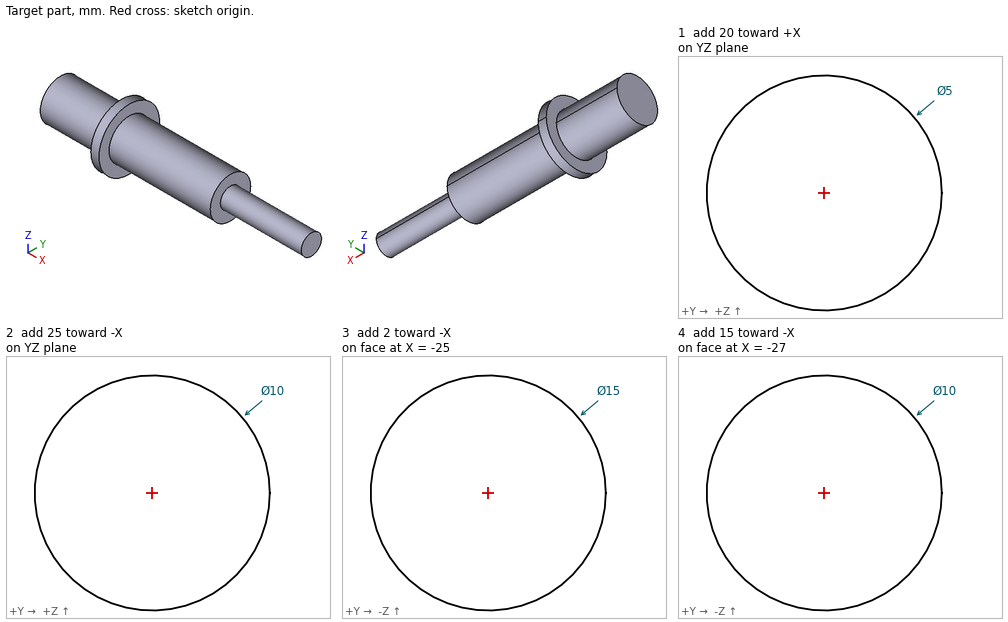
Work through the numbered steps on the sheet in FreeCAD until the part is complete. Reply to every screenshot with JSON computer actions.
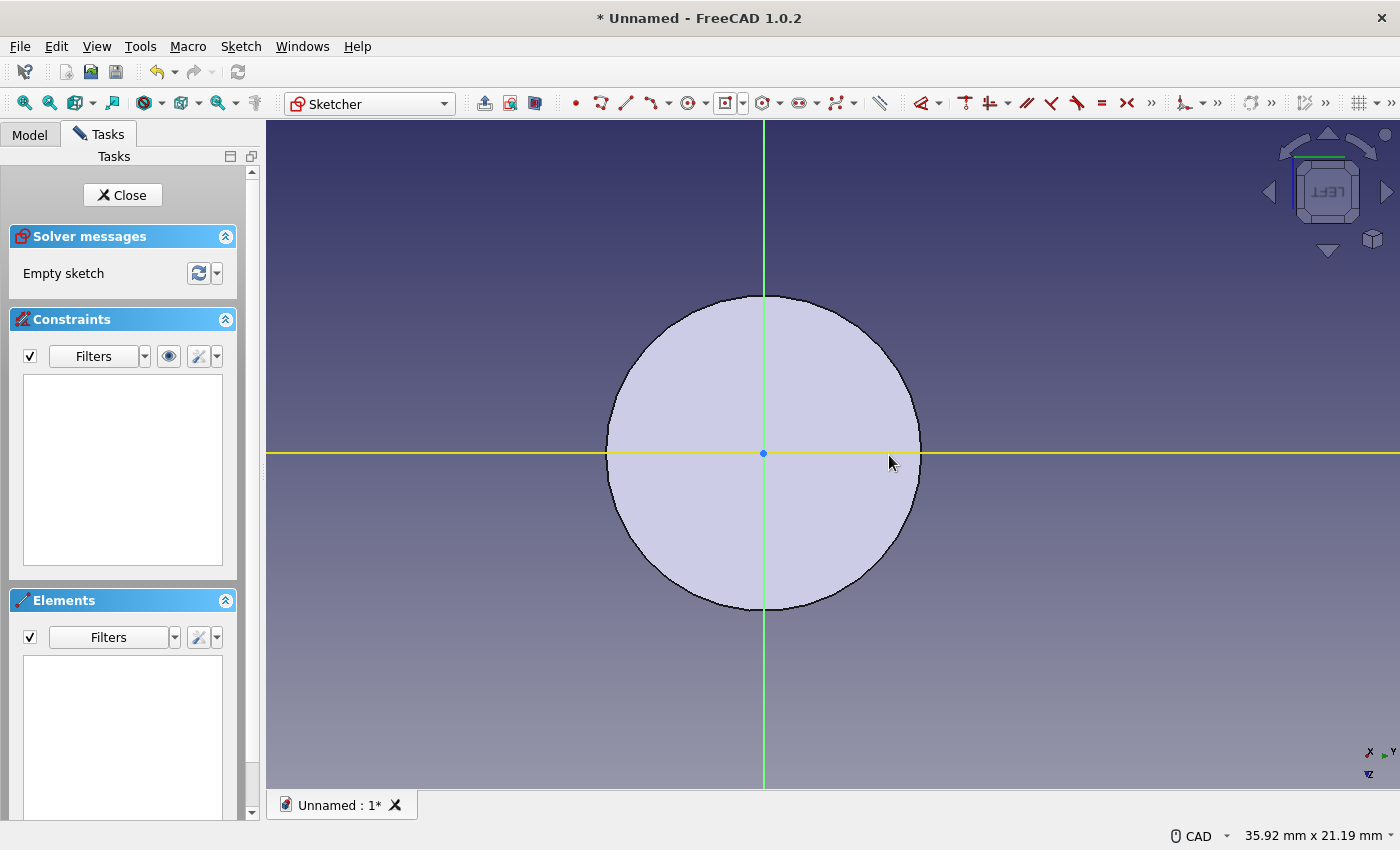
{"action": "key", "text": "g c"}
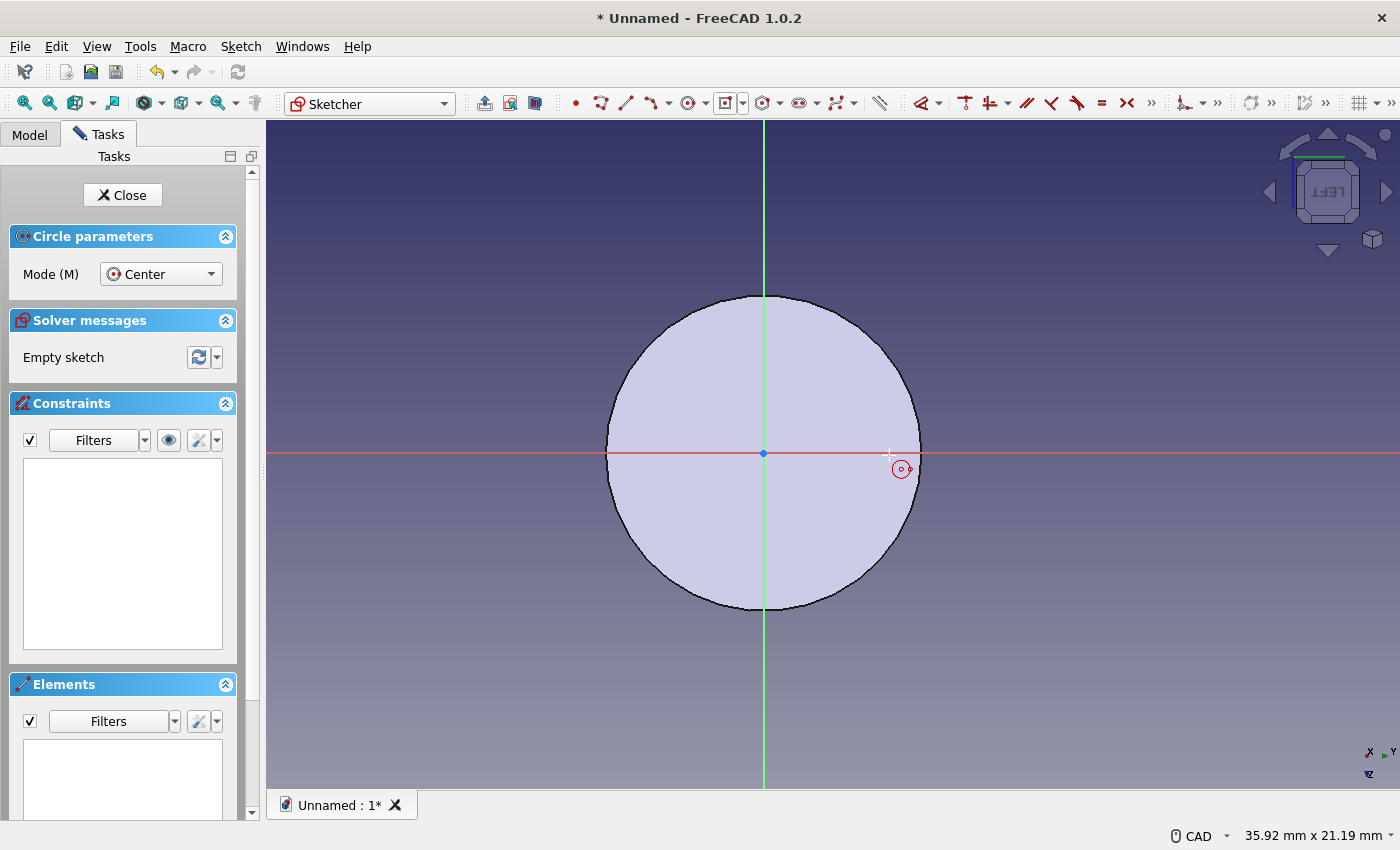
{"action": "left_click", "coordinate": [764, 453]}
{"action": "left_click", "coordinate": [931, 286]}
{"action": "key", "text": "Escape"}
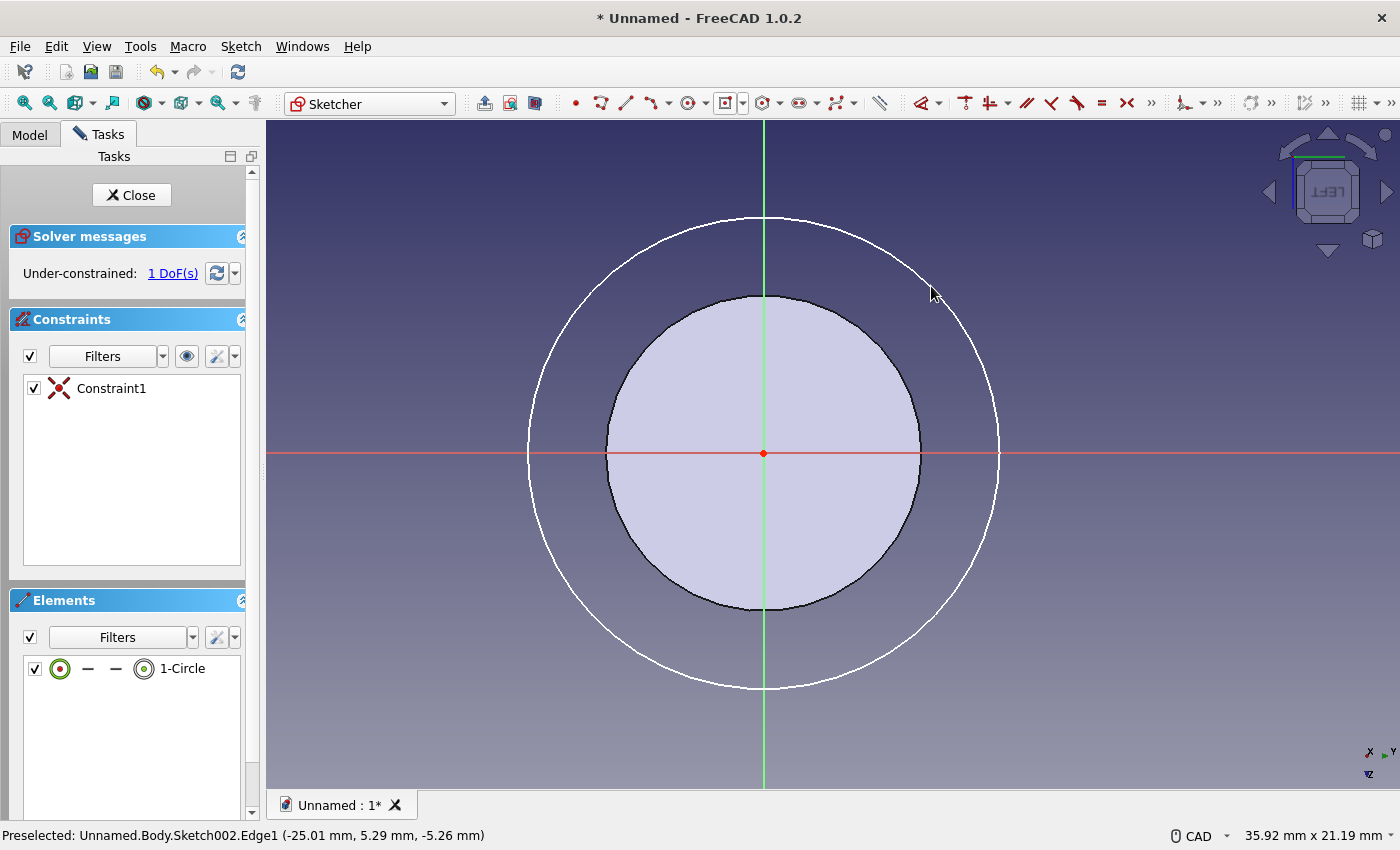
{"action": "key", "text": "d"}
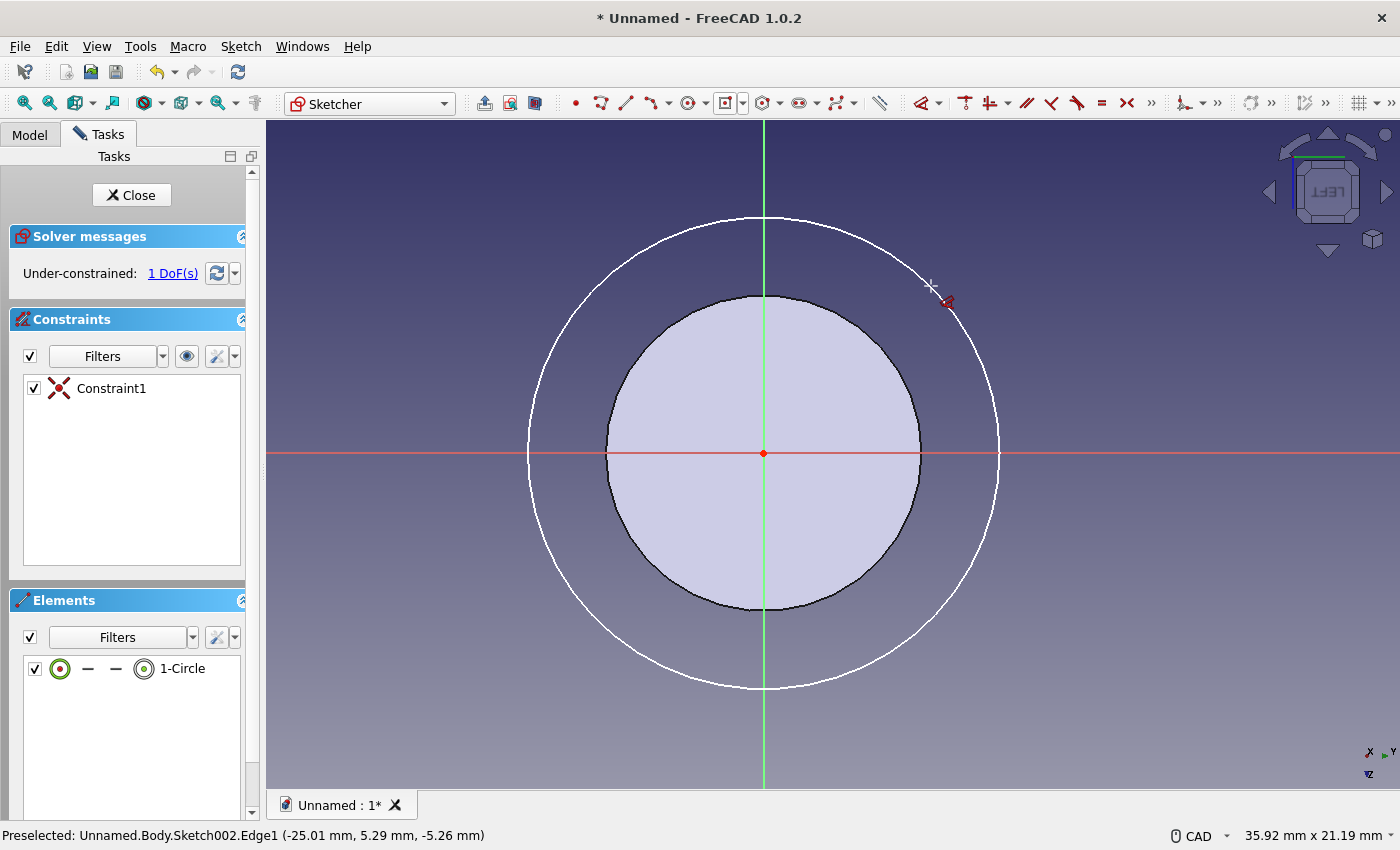
{"action": "left_click", "coordinate": [930, 286]}
{"action": "left_click", "coordinate": [953, 263]}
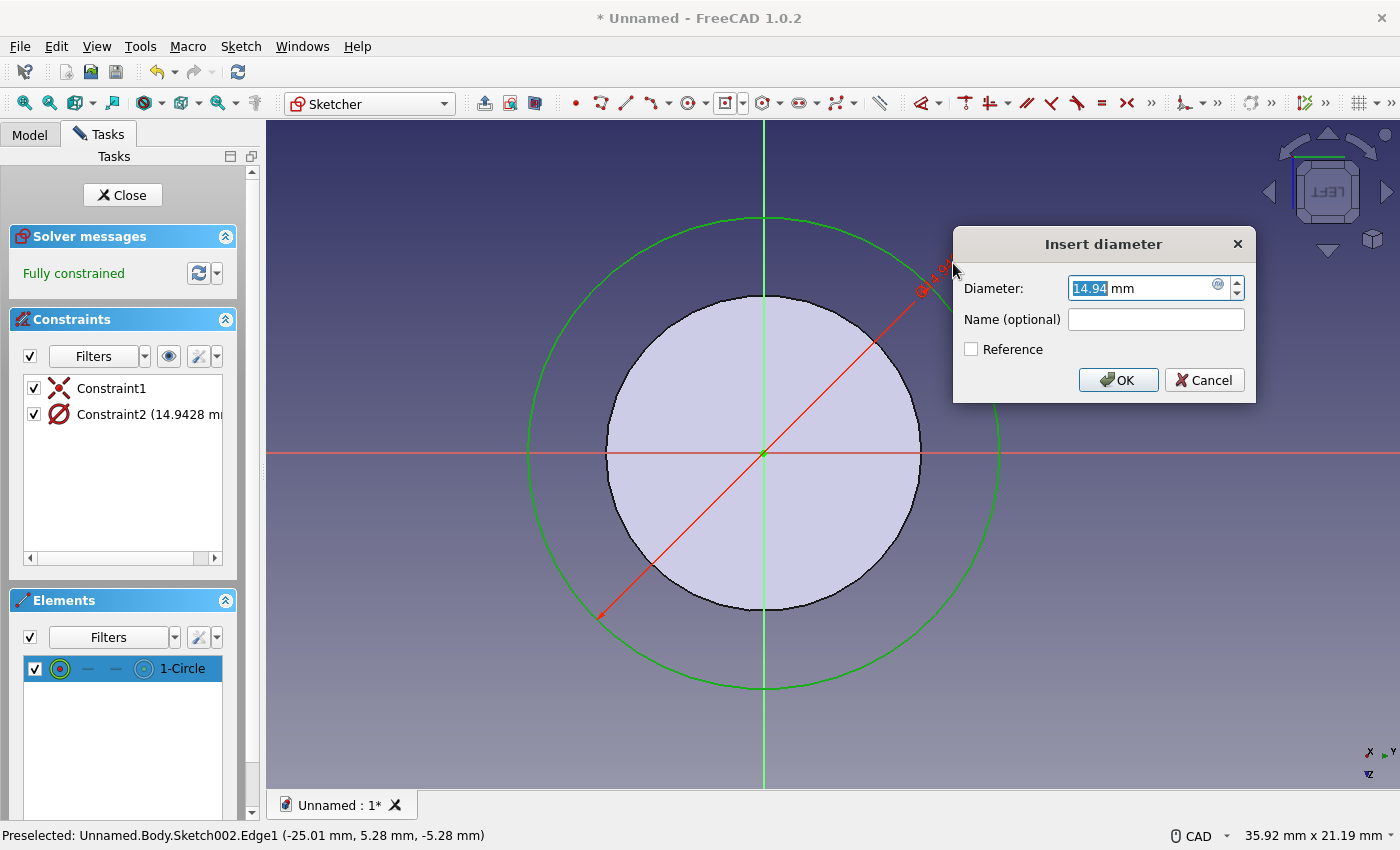
{"action": "type", "text": "15"}
{"action": "key", "text": "Return"}
{"action": "key", "text": "Escape"}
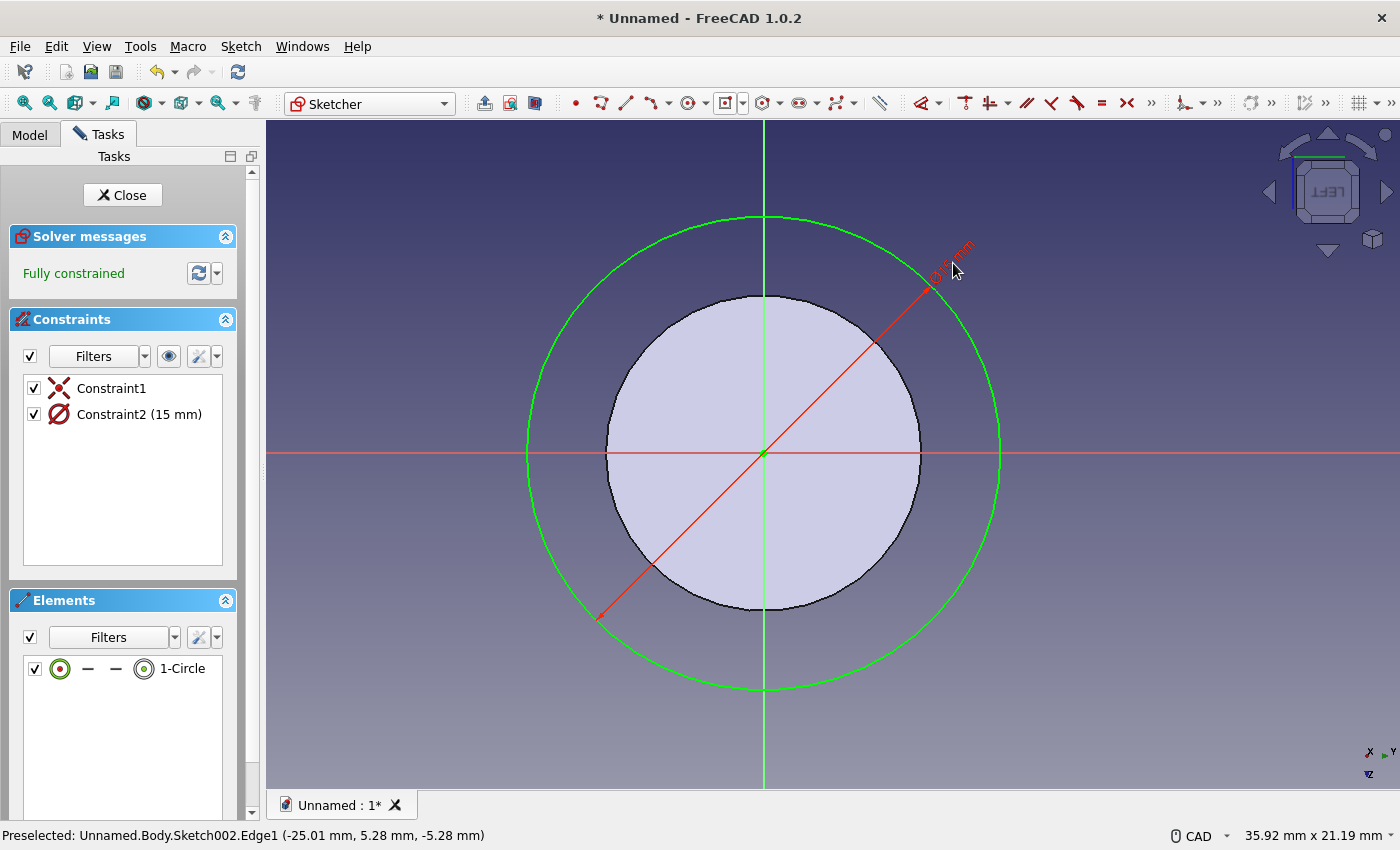
{"action": "left_click", "coordinate": [123, 195]}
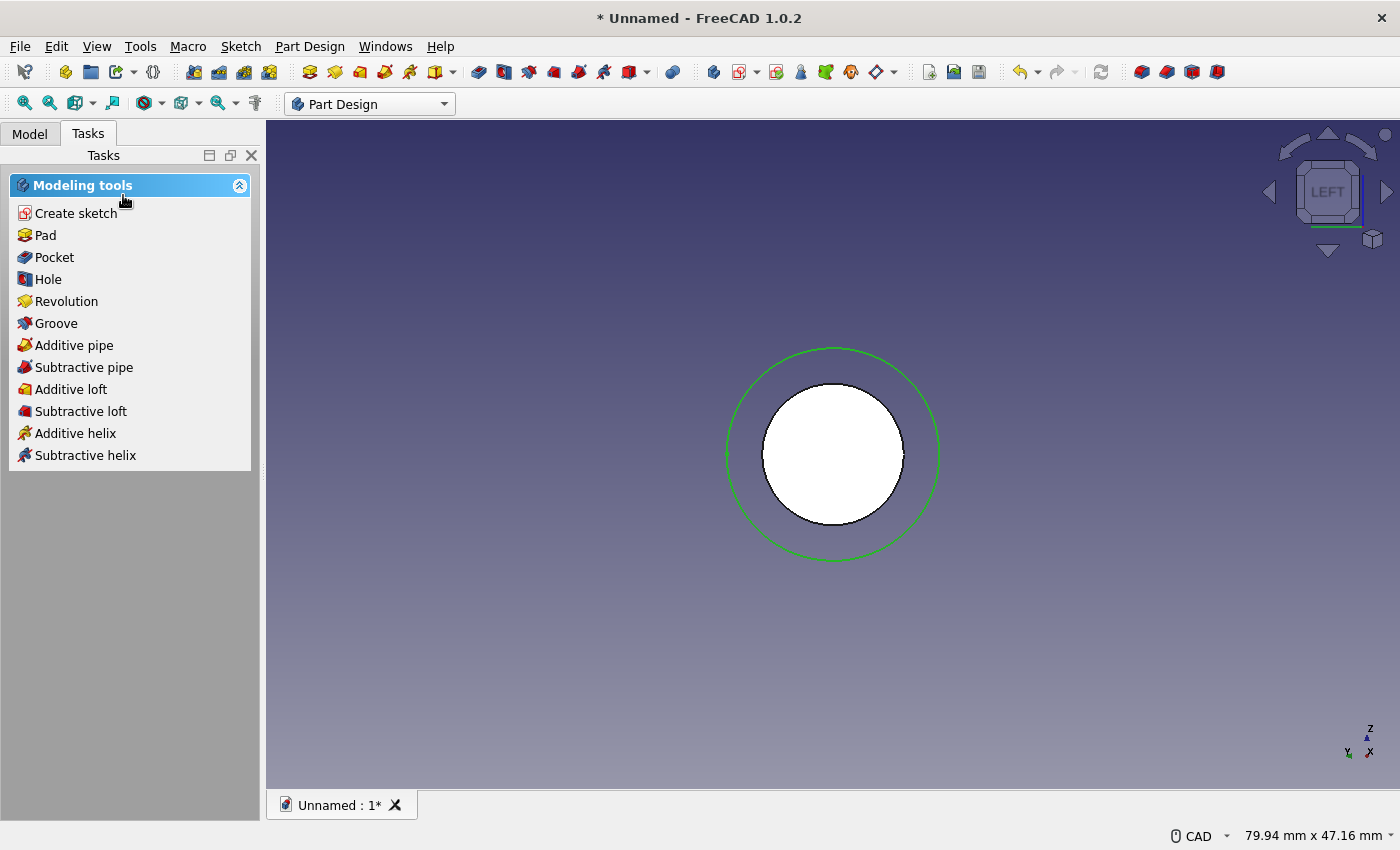
{"action": "left_click", "coordinate": [310, 72]}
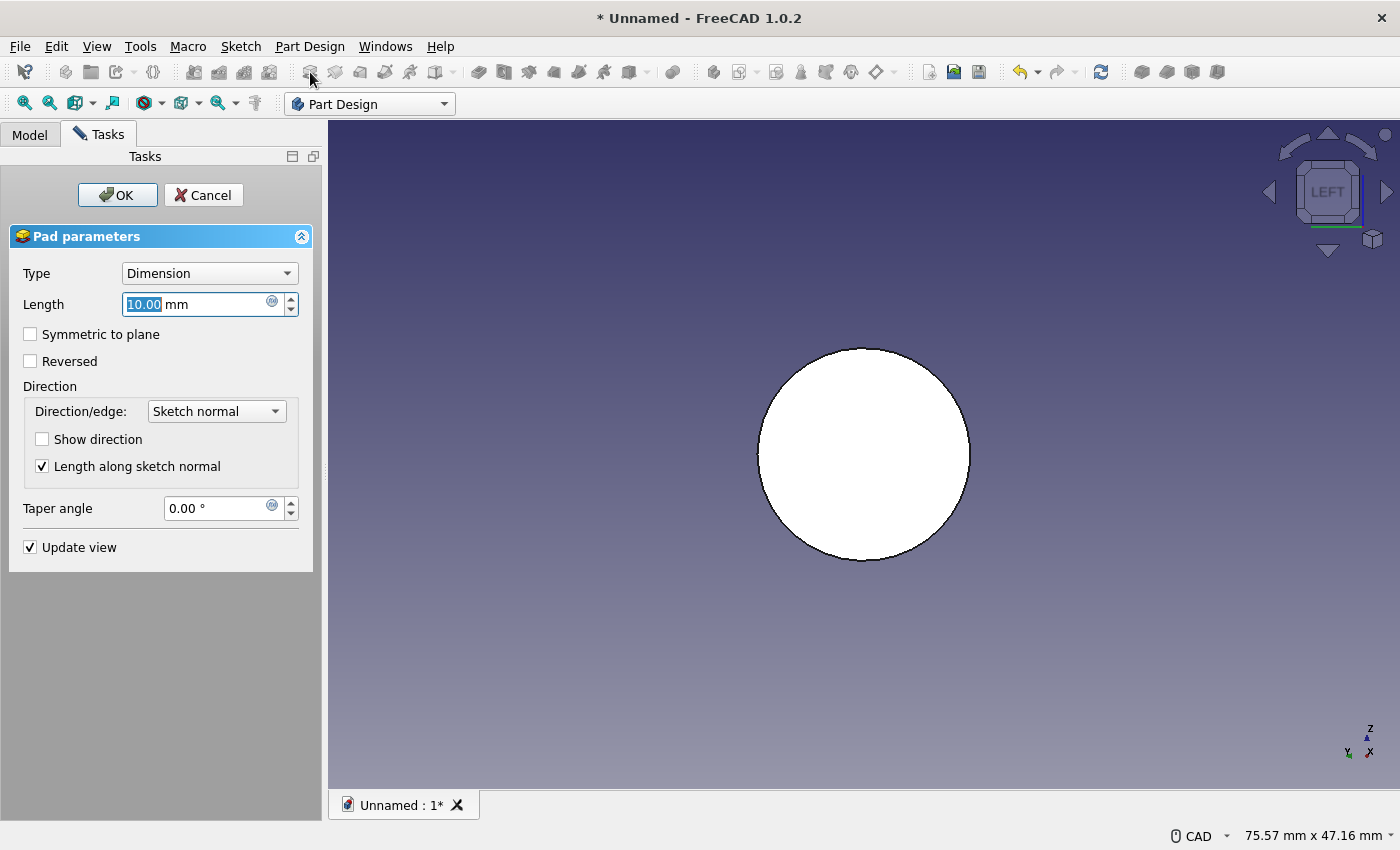
{"action": "type", "text": "2"}
{"action": "key", "text": "Tab"}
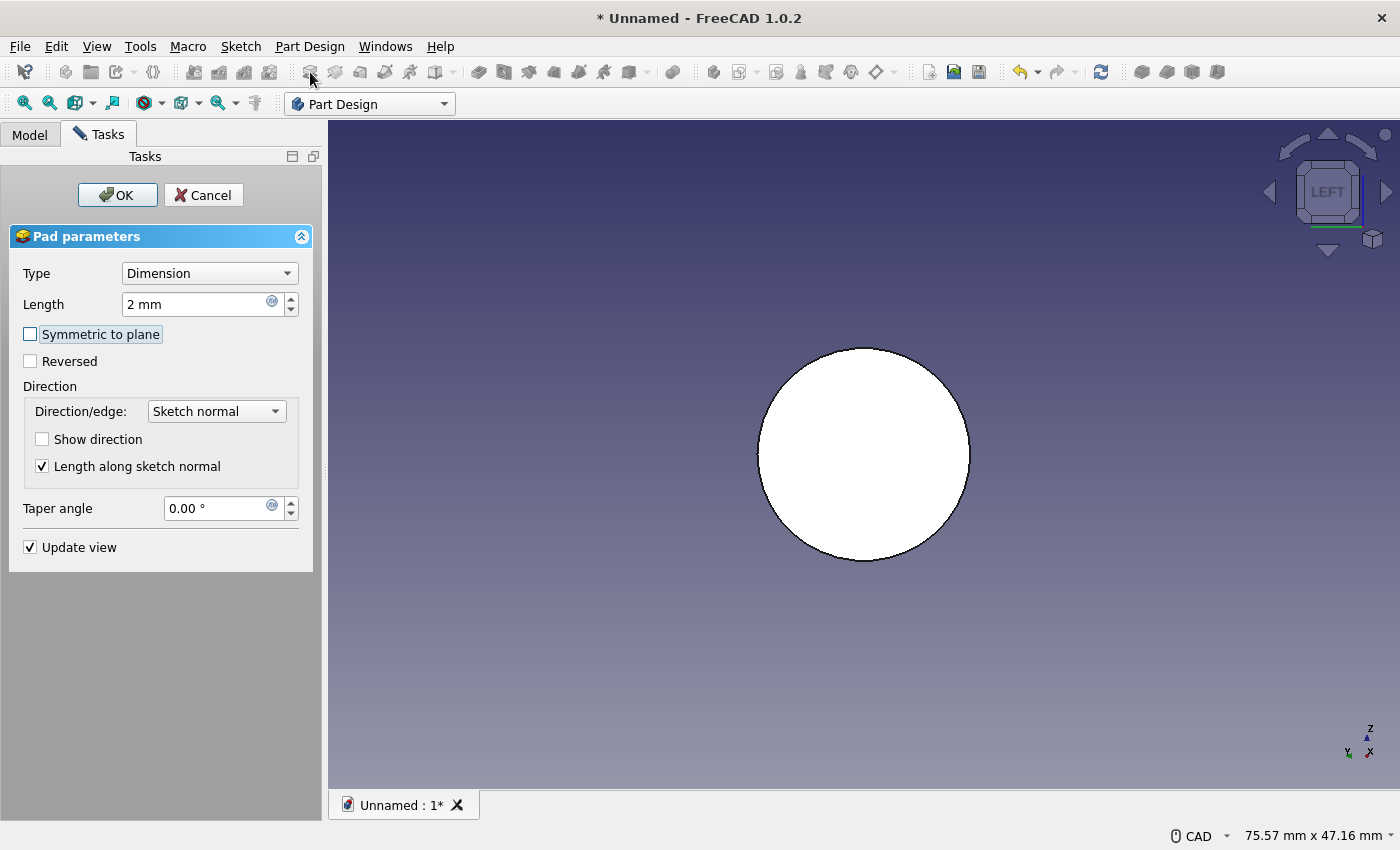
{"action": "left_click", "coordinate": [118, 195]}